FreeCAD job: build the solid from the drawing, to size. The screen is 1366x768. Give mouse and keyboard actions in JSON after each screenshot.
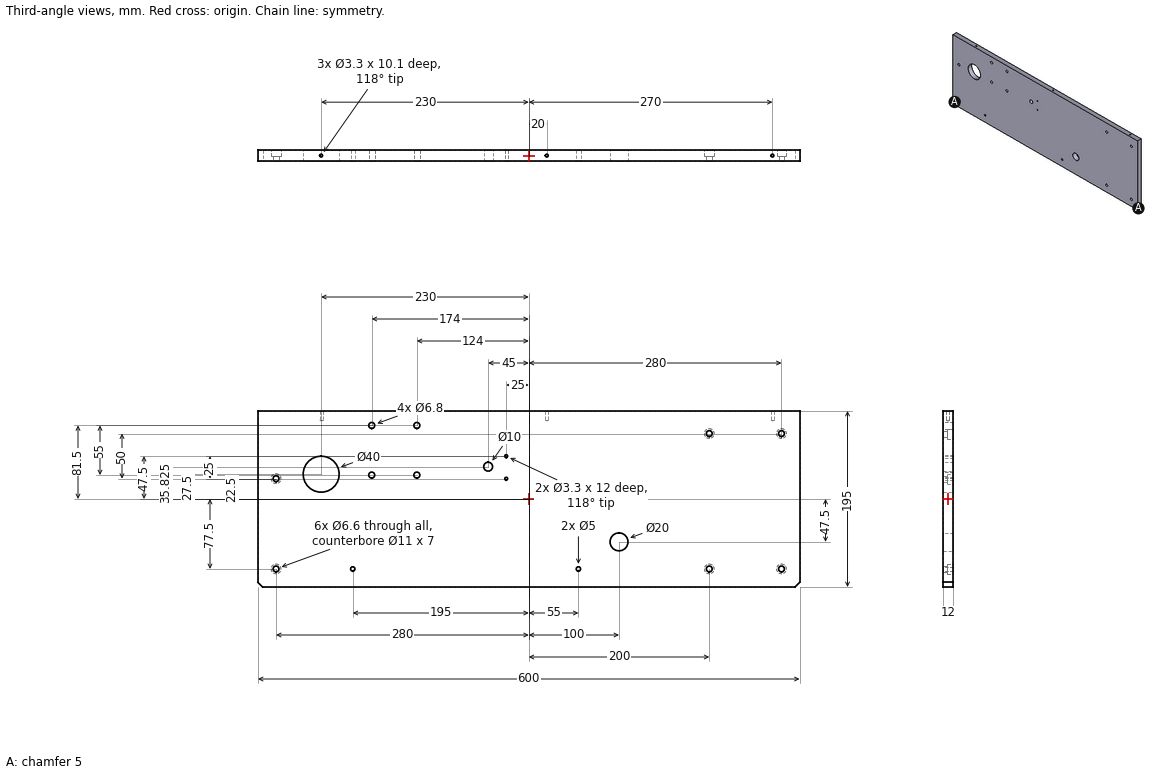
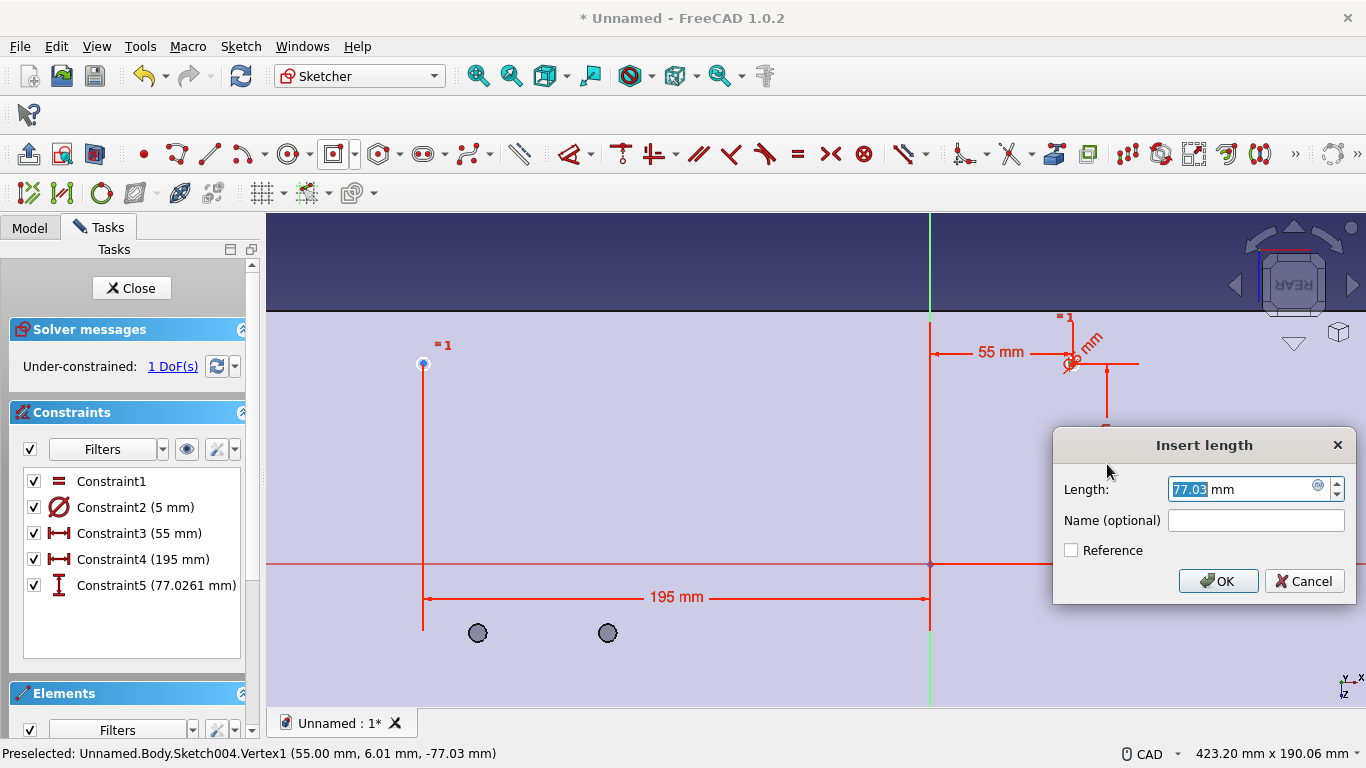
{"action": "type", "text": "77.5"}
{"action": "key", "text": "Return"}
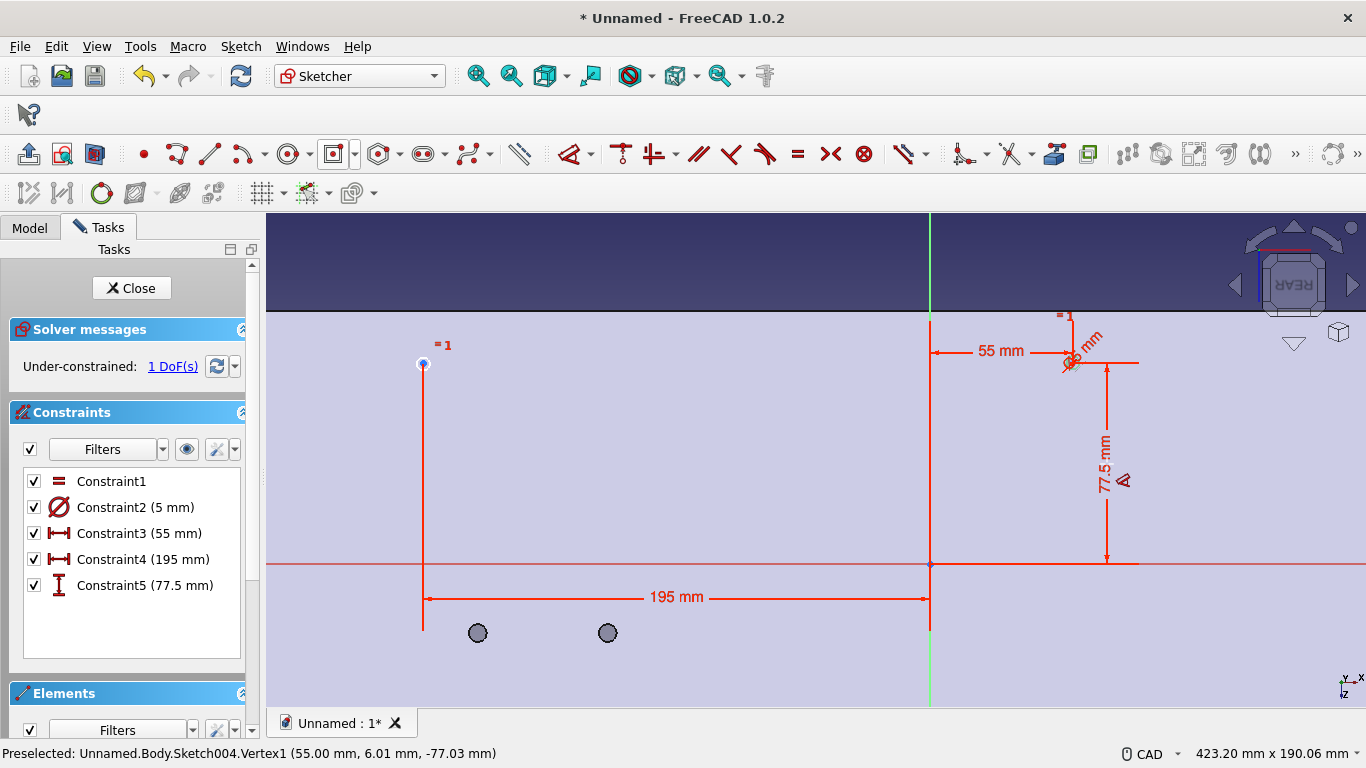
{"action": "left_click", "coordinate": [423, 364]}
{"action": "left_click", "coordinate": [389, 464]}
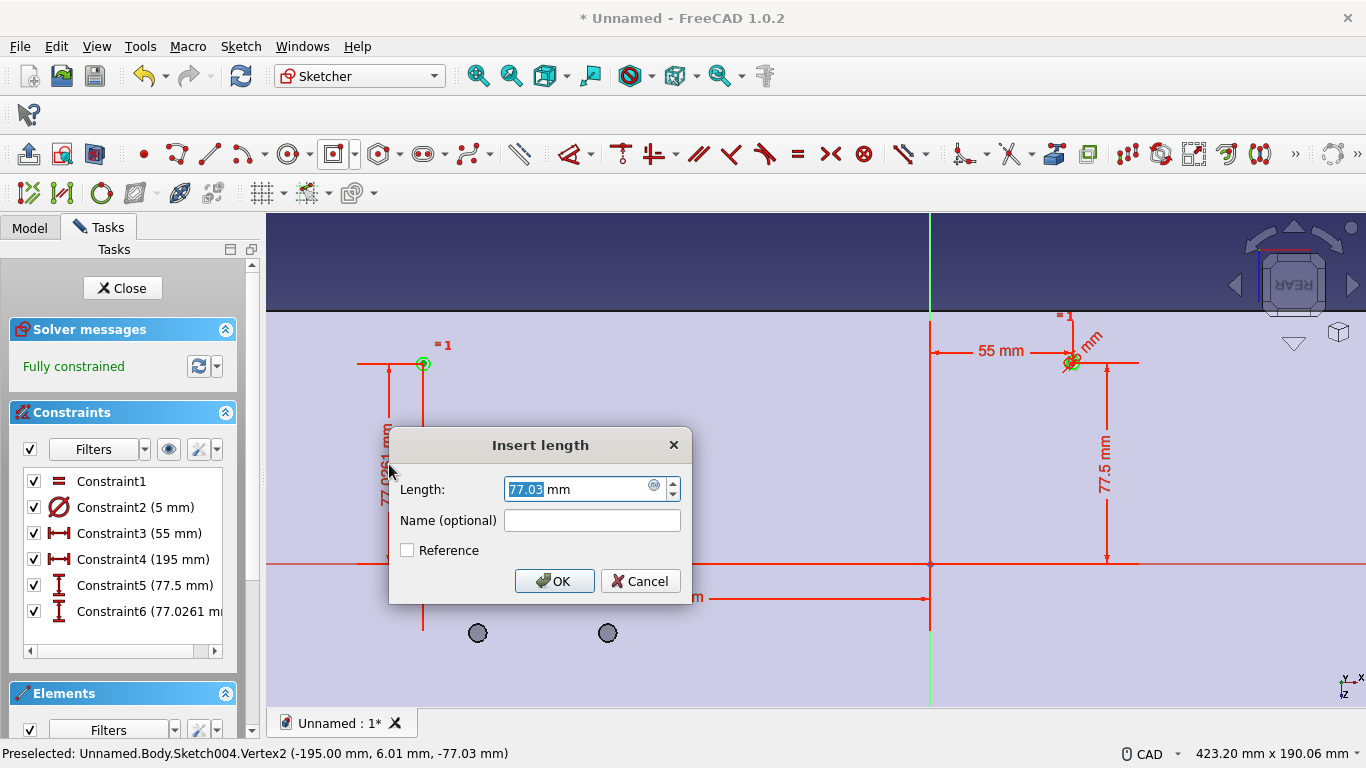
{"action": "type", "text": "77.5"}
{"action": "key", "text": "Return"}
{"action": "key", "text": "Escape"}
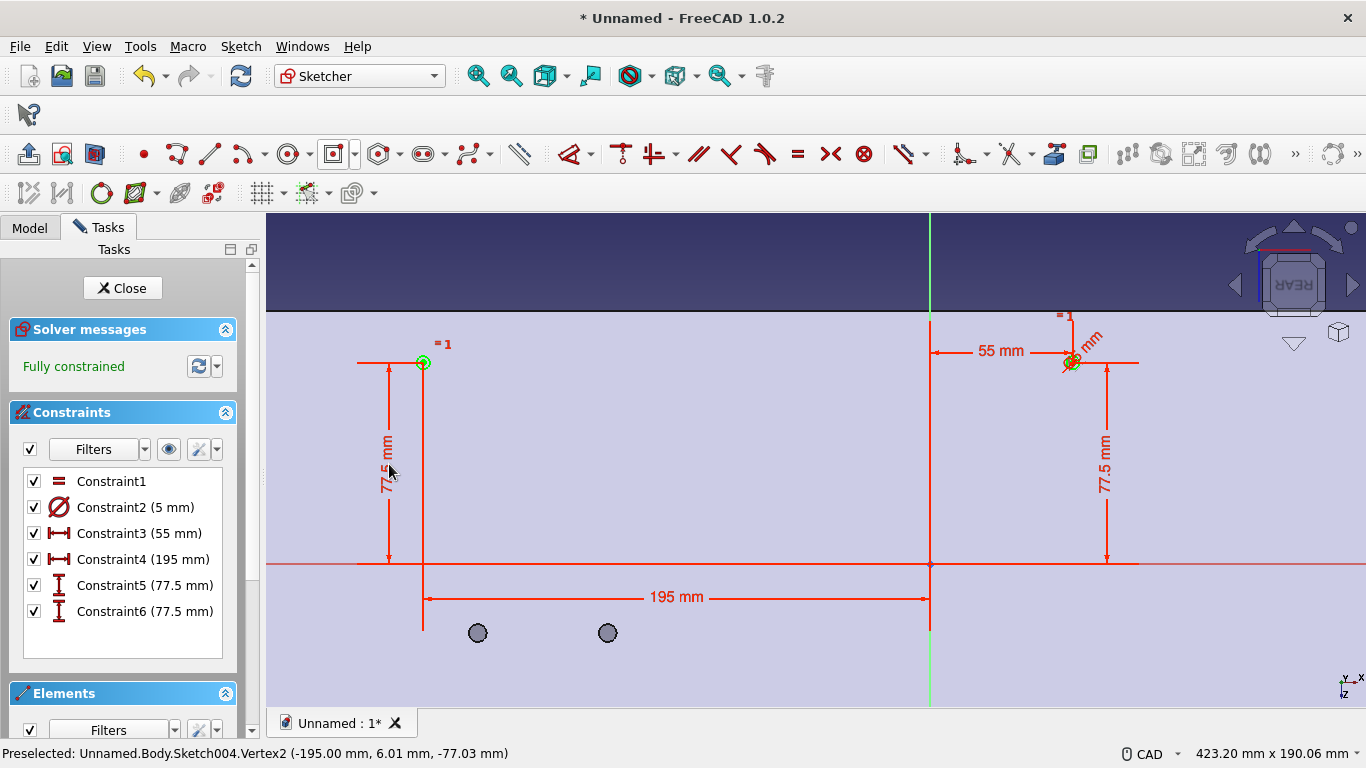
{"action": "left_click", "coordinate": [123, 288]}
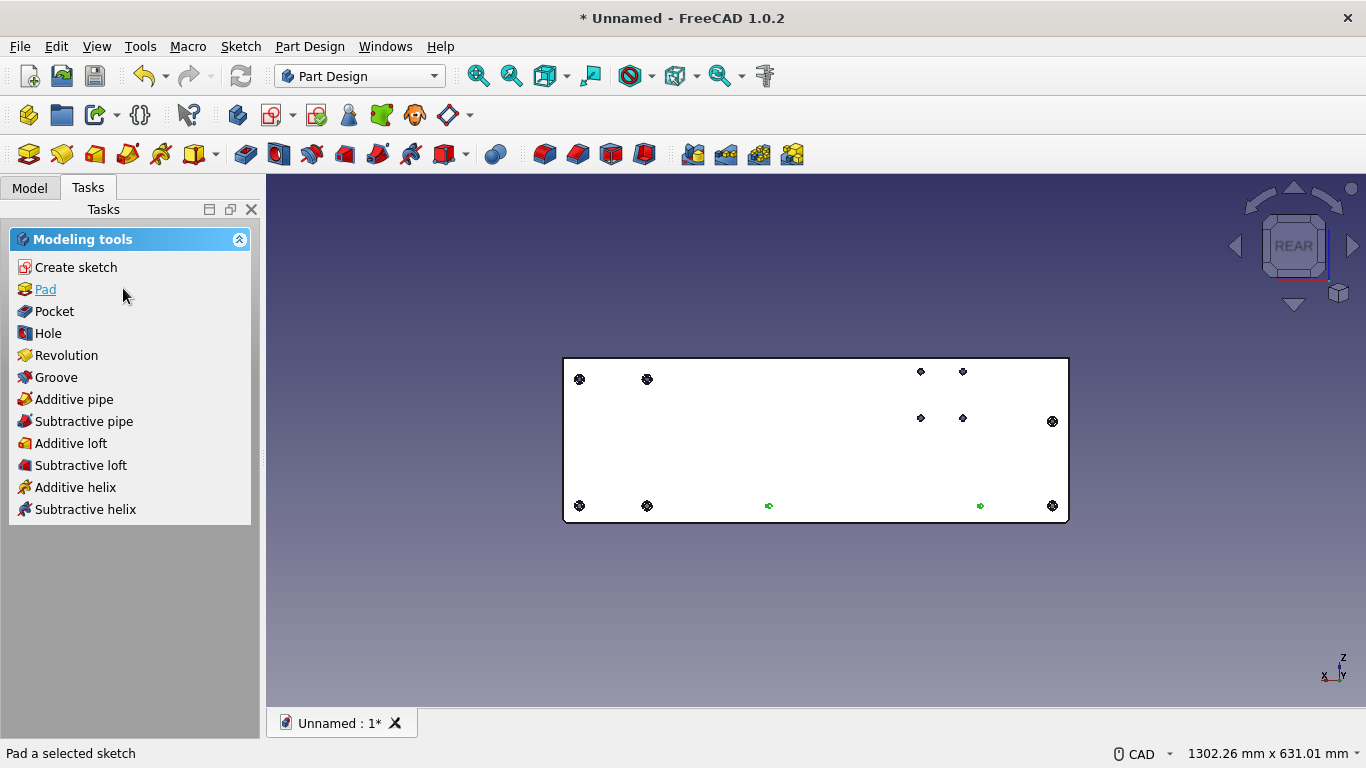
{"action": "left_click", "coordinate": [246, 154]}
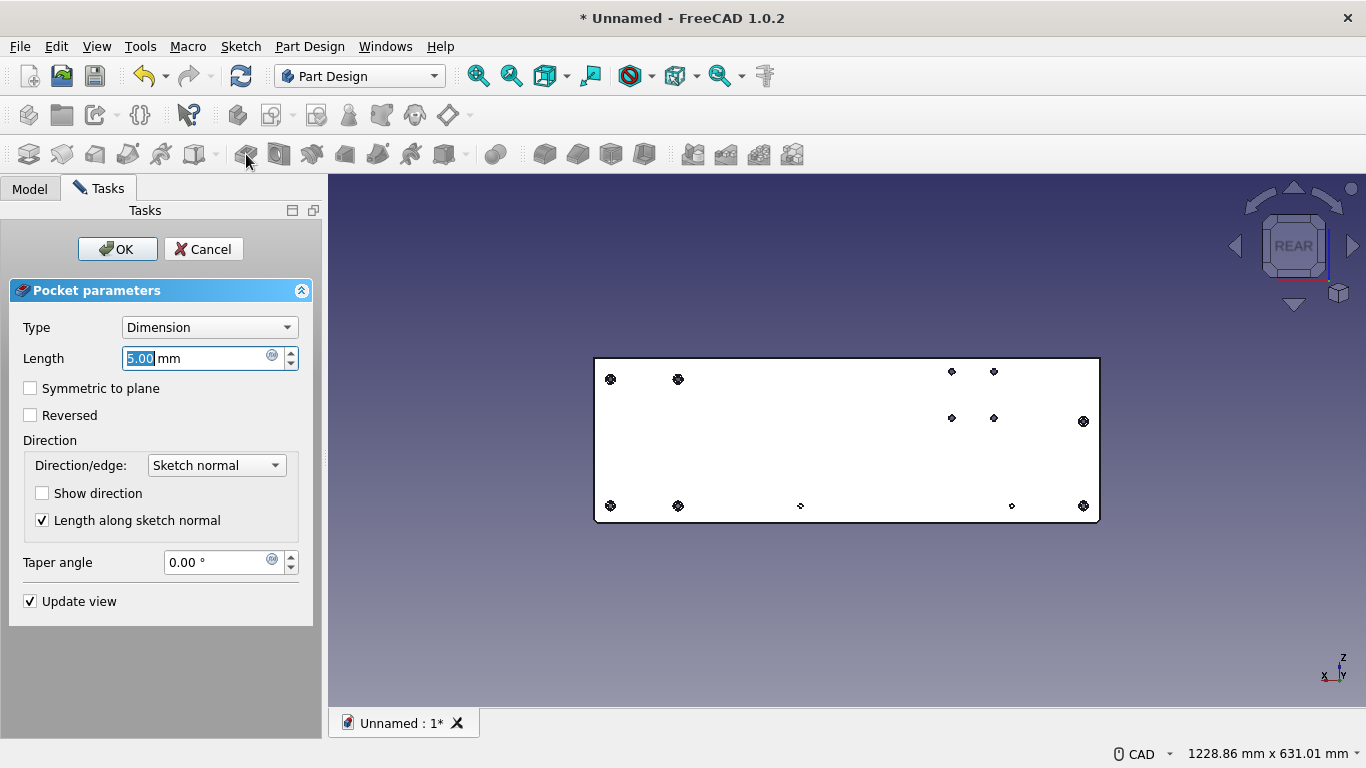
{"action": "left_click", "coordinate": [210, 328]}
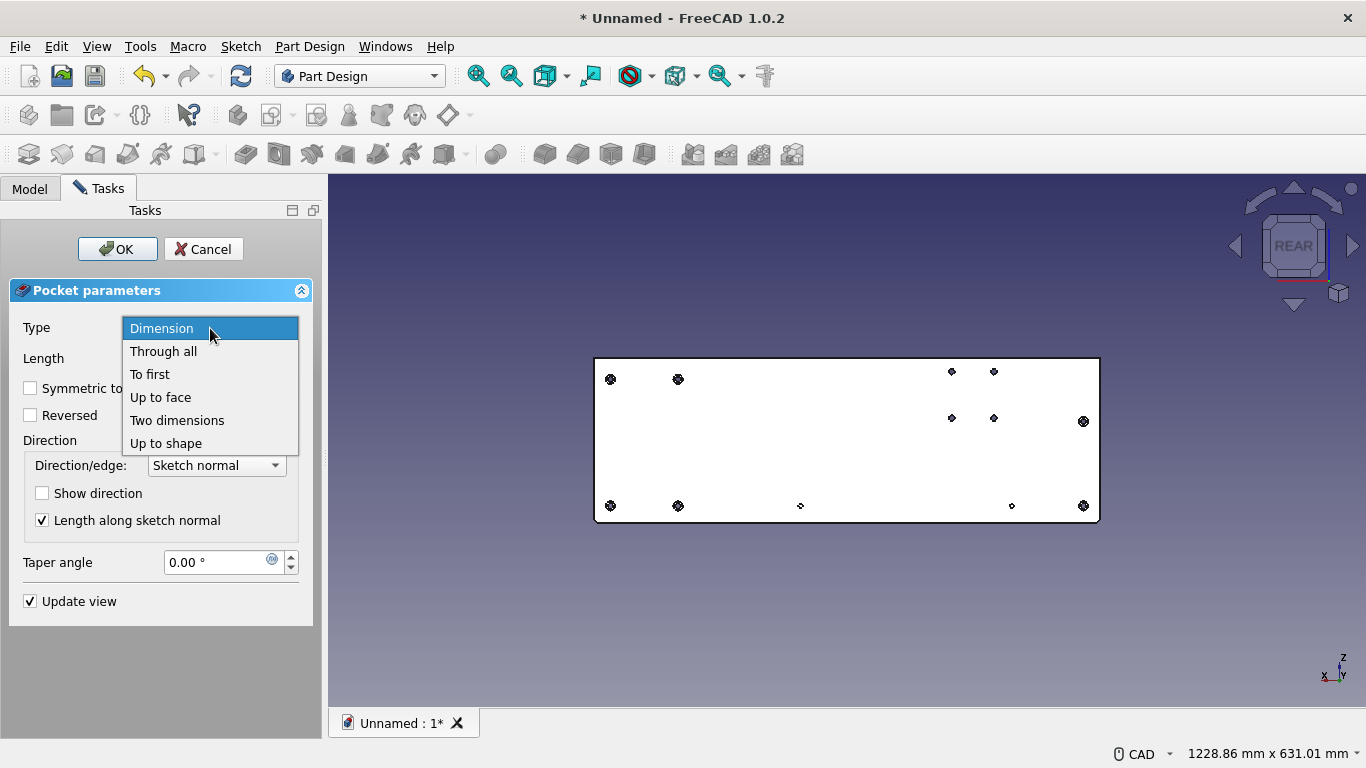
{"action": "left_click", "coordinate": [208, 352]}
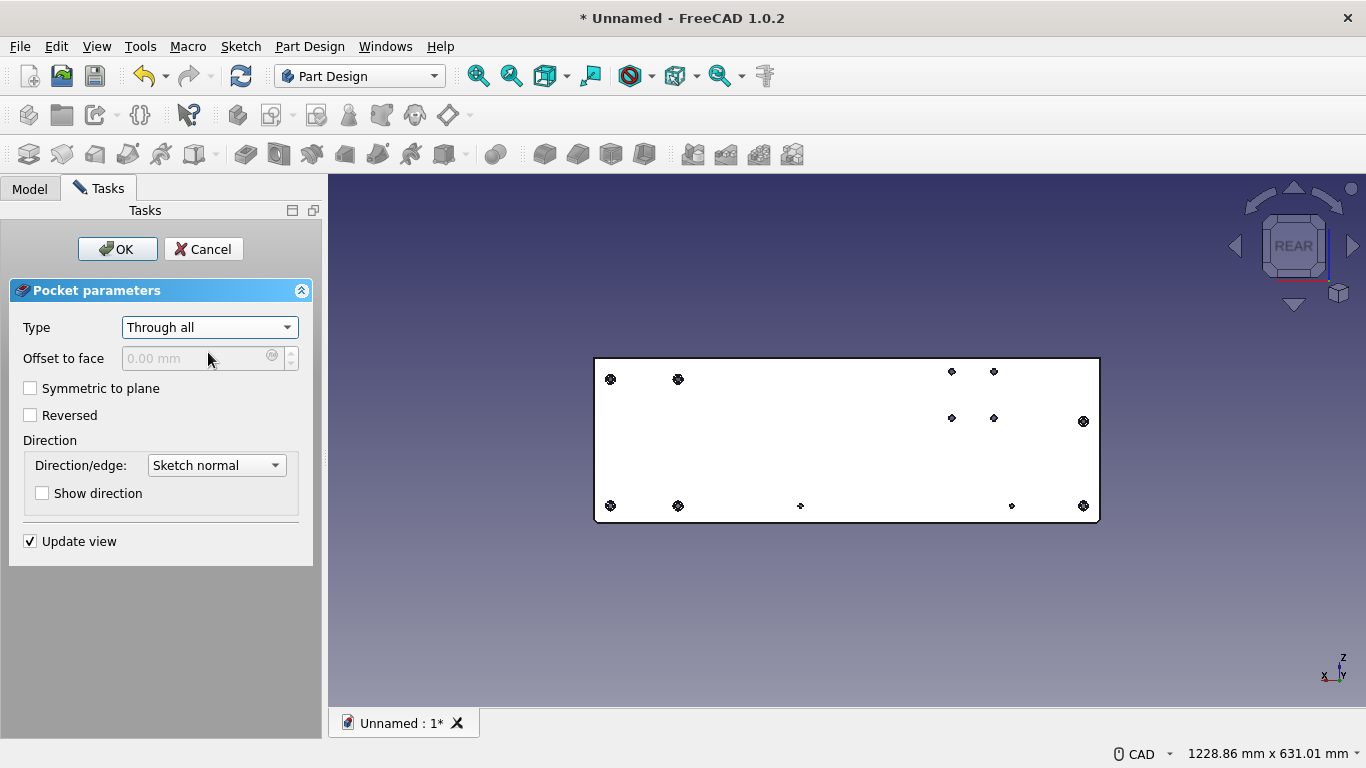
{"action": "left_click", "coordinate": [118, 249]}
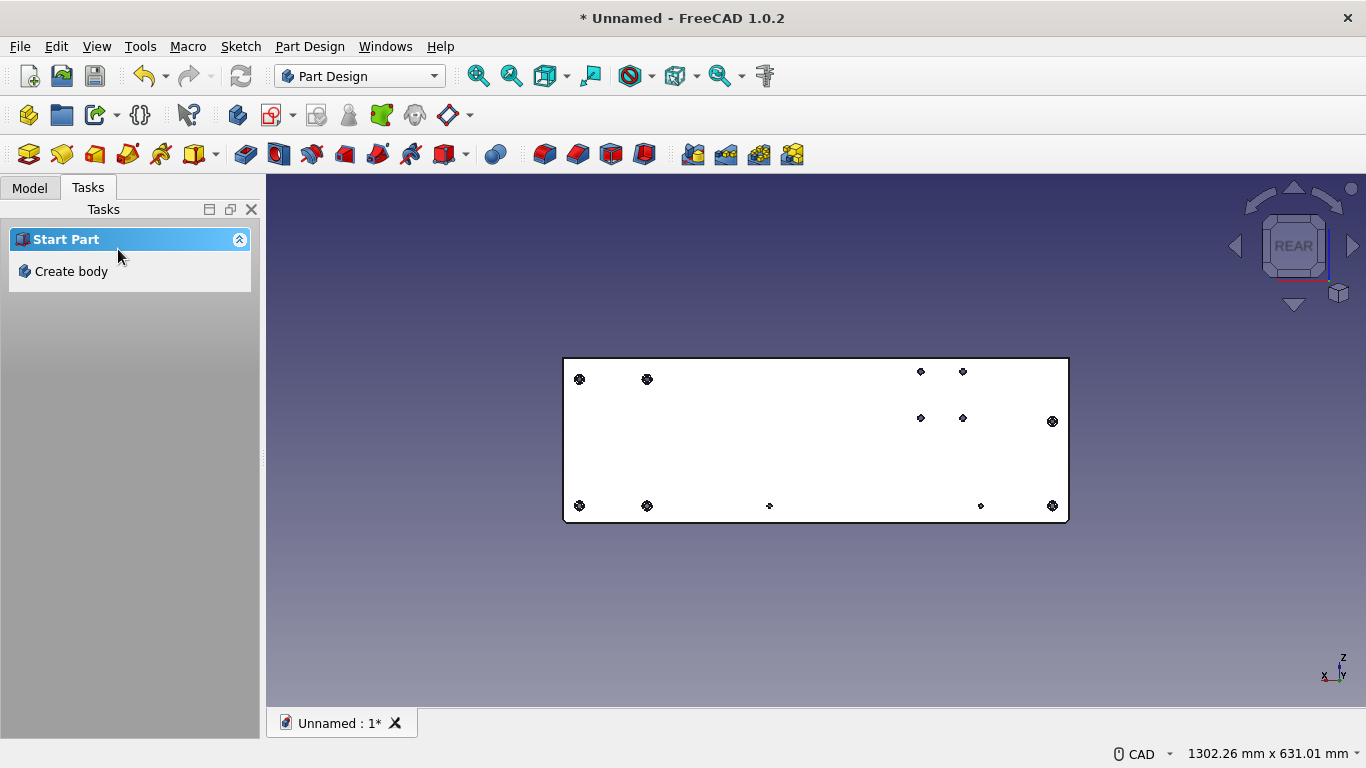
{"action": "left_click", "coordinate": [816, 439]}